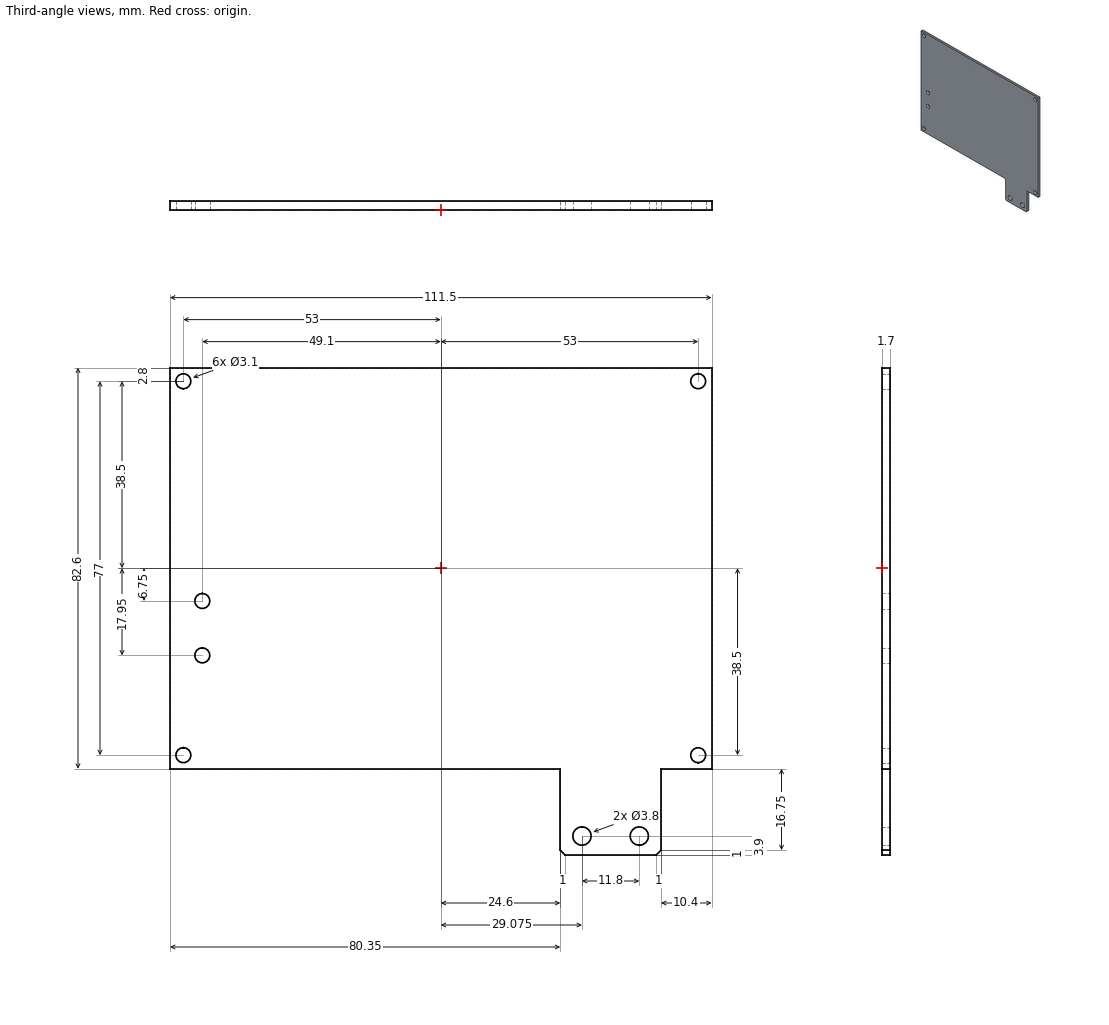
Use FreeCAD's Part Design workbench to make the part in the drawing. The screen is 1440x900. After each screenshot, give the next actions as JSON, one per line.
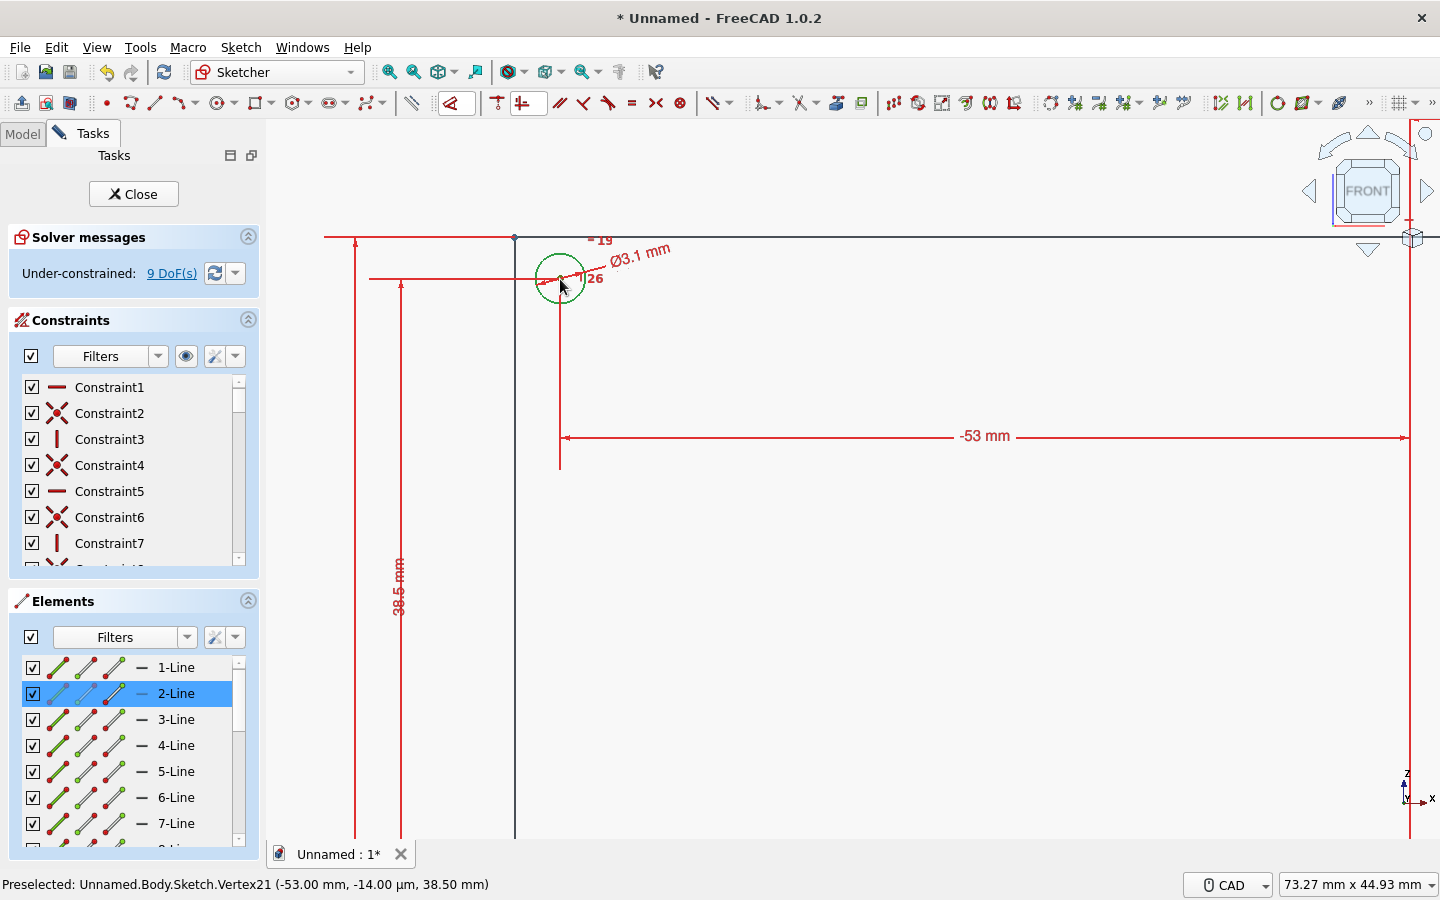
{"action": "key", "text": "i"}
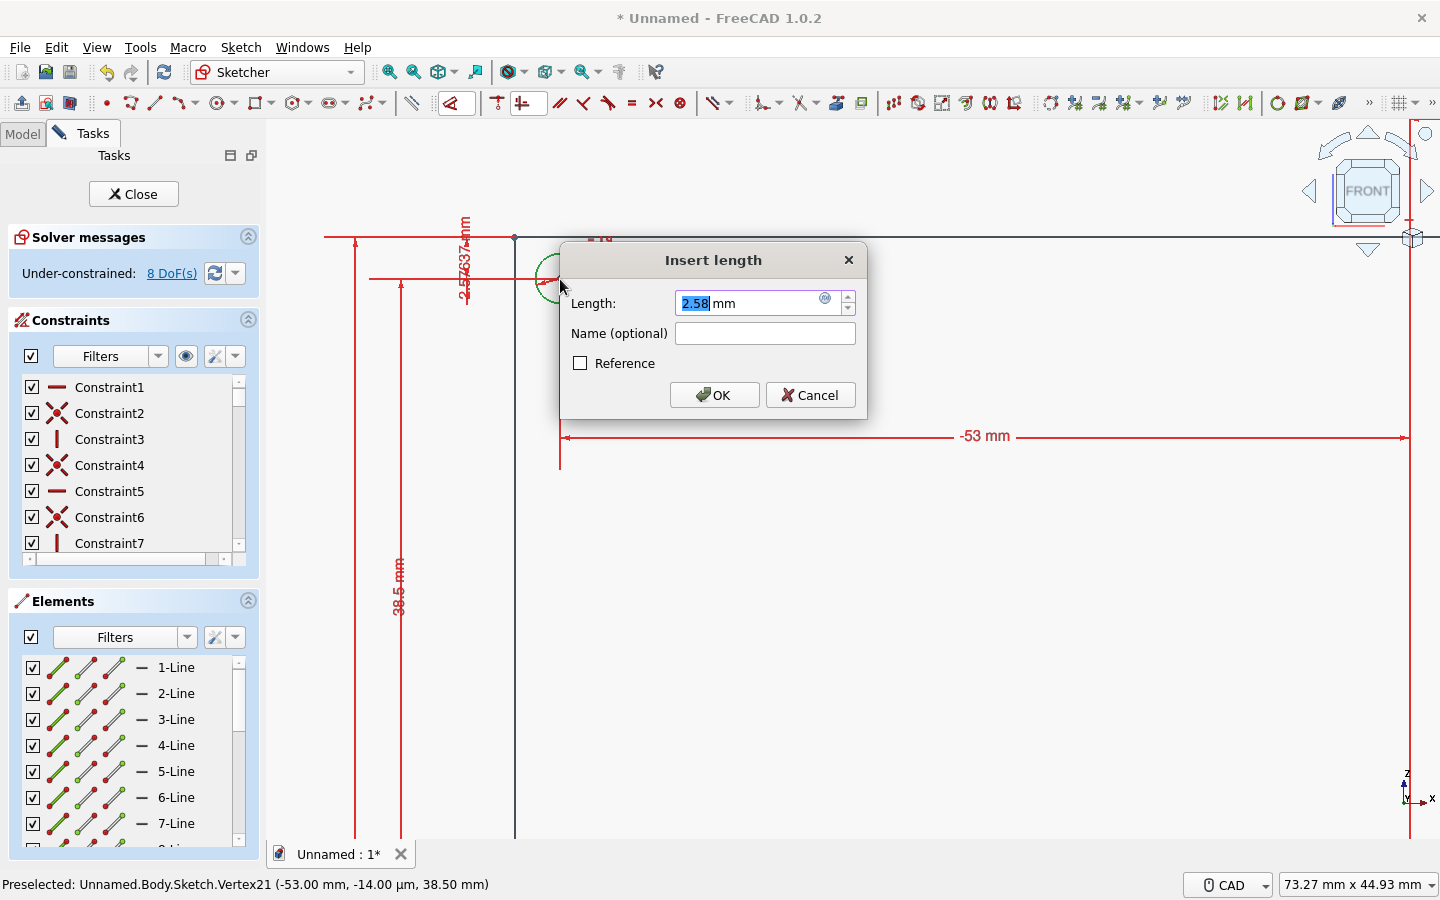
{"action": "type", "text": "2.8"}
{"action": "key", "text": "Return"}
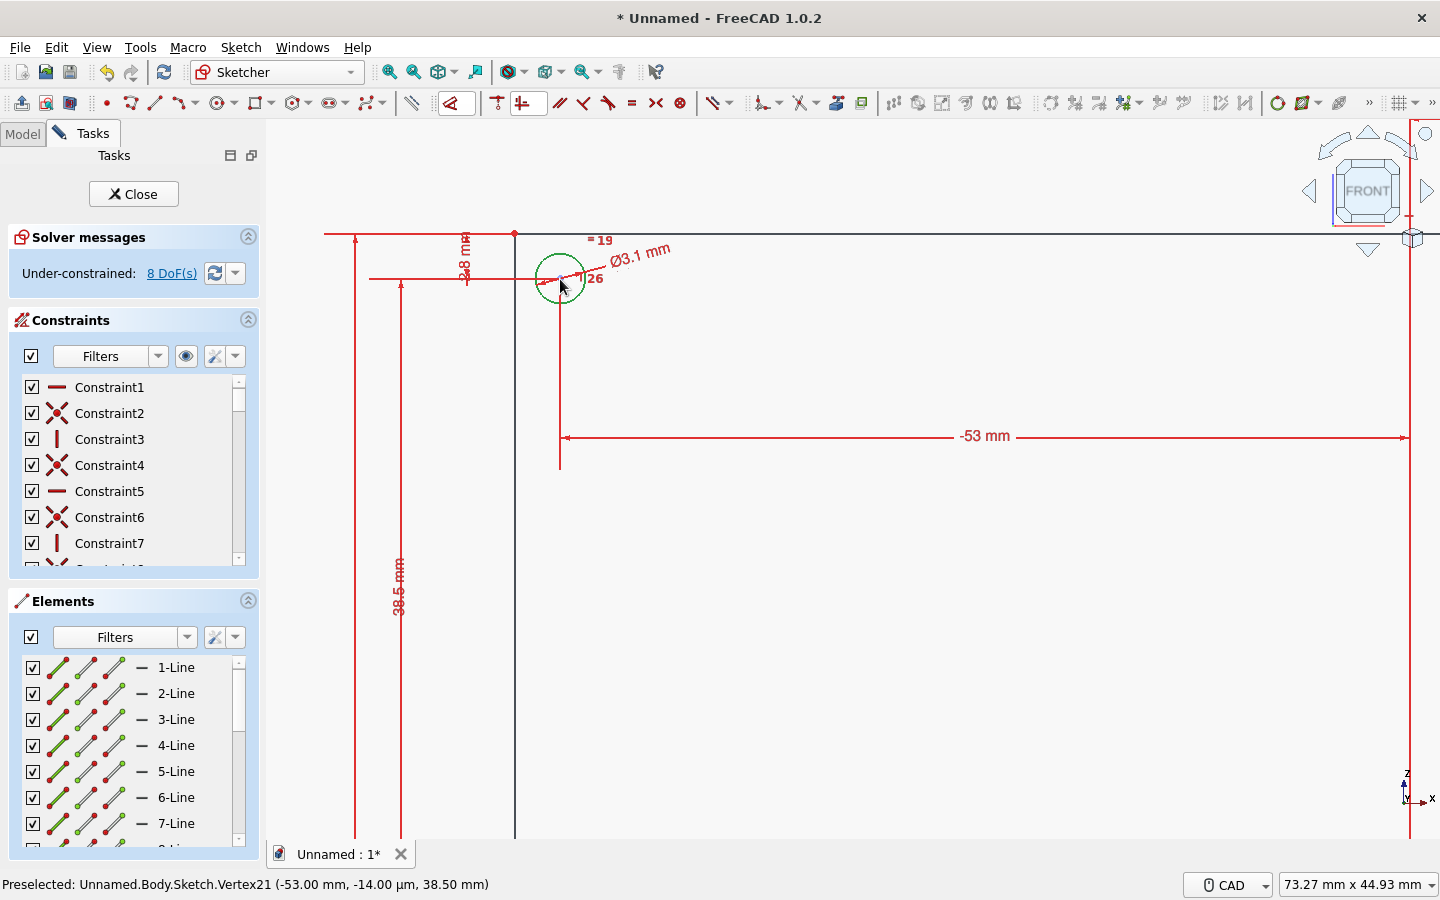
{"action": "scroll", "coordinate": [515, 238], "scroll_direction": "down", "scroll_amount": 6}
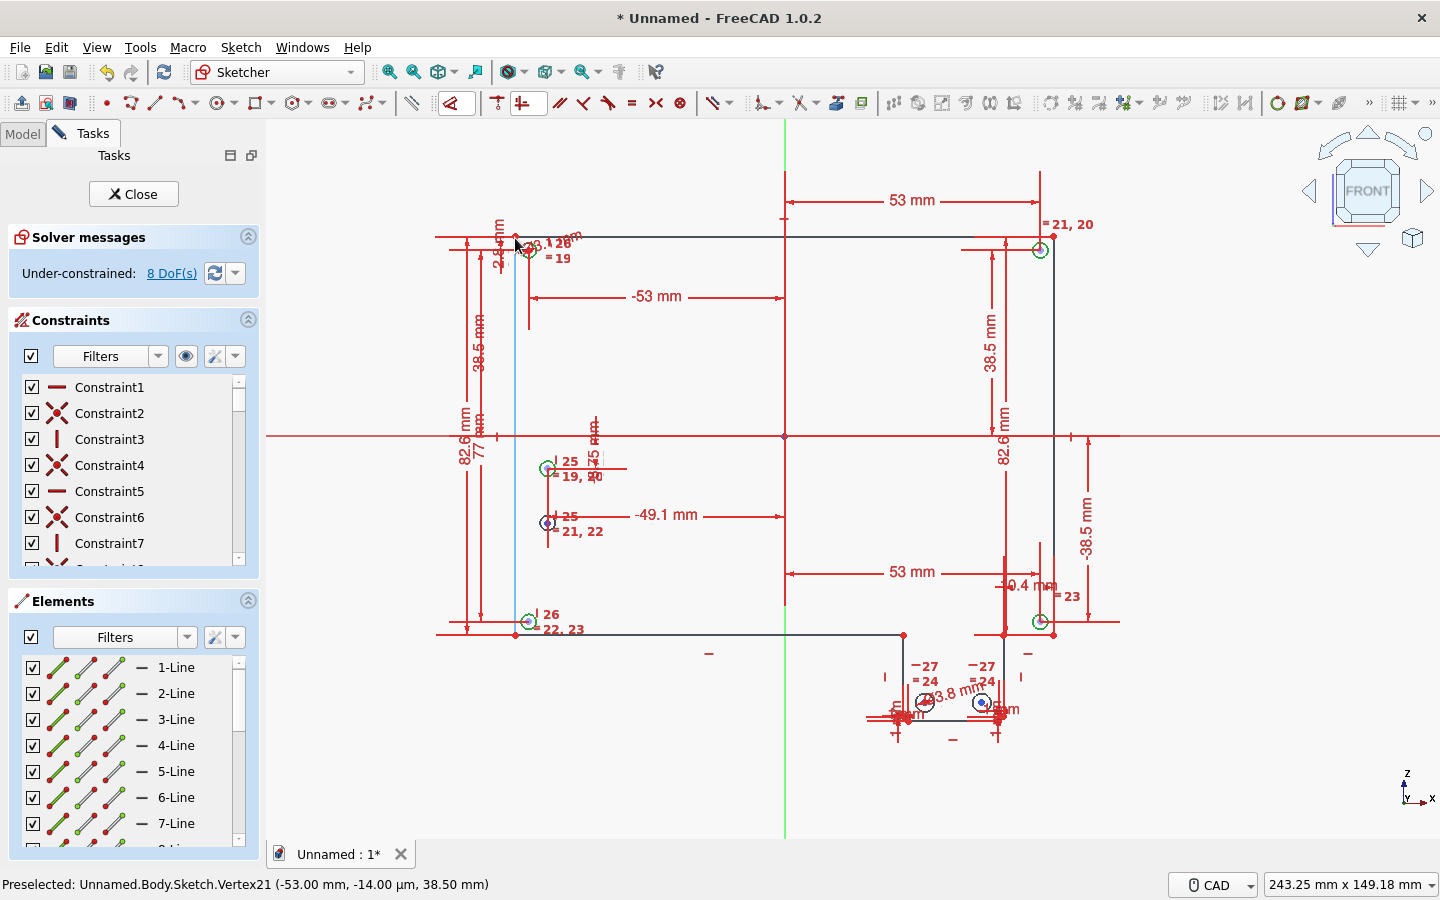
{"action": "scroll", "coordinate": [908, 721], "scroll_direction": "up", "scroll_amount": 4}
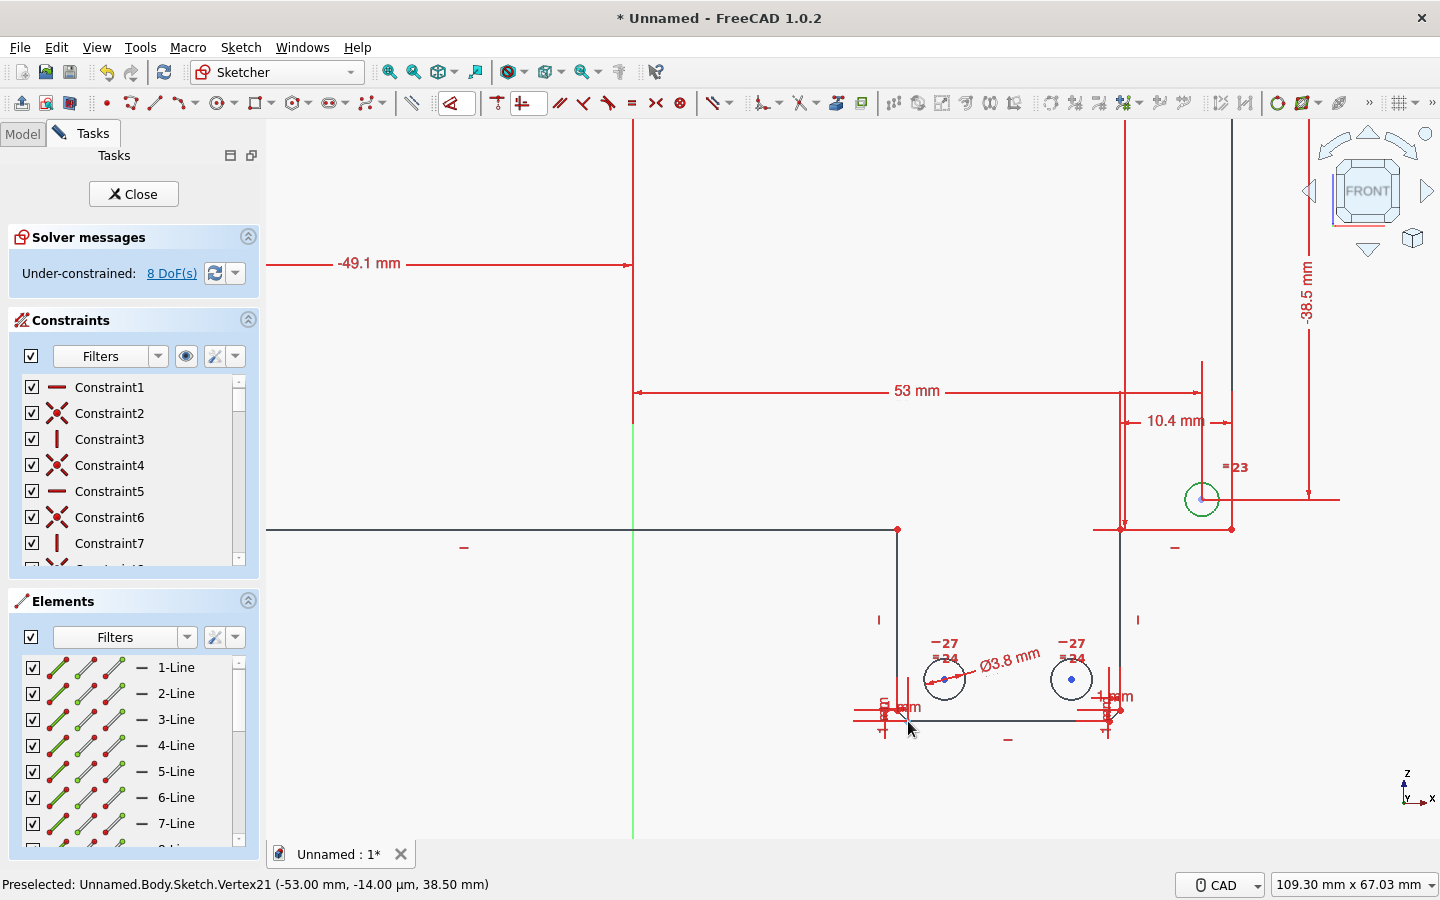
{"action": "left_click", "coordinate": [908, 721]}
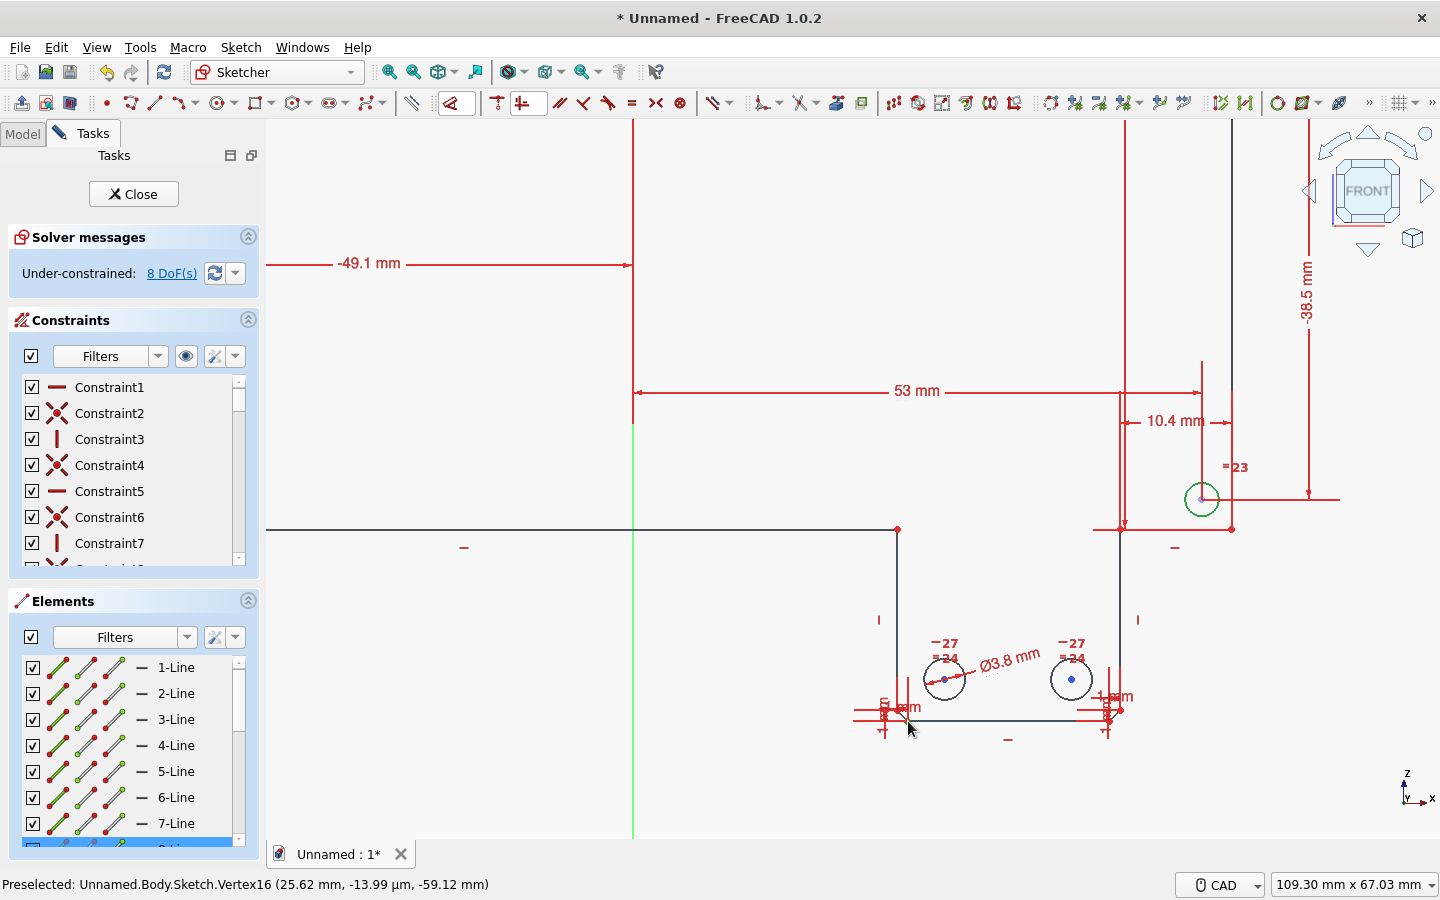
{"action": "left_click", "coordinate": [945, 679]}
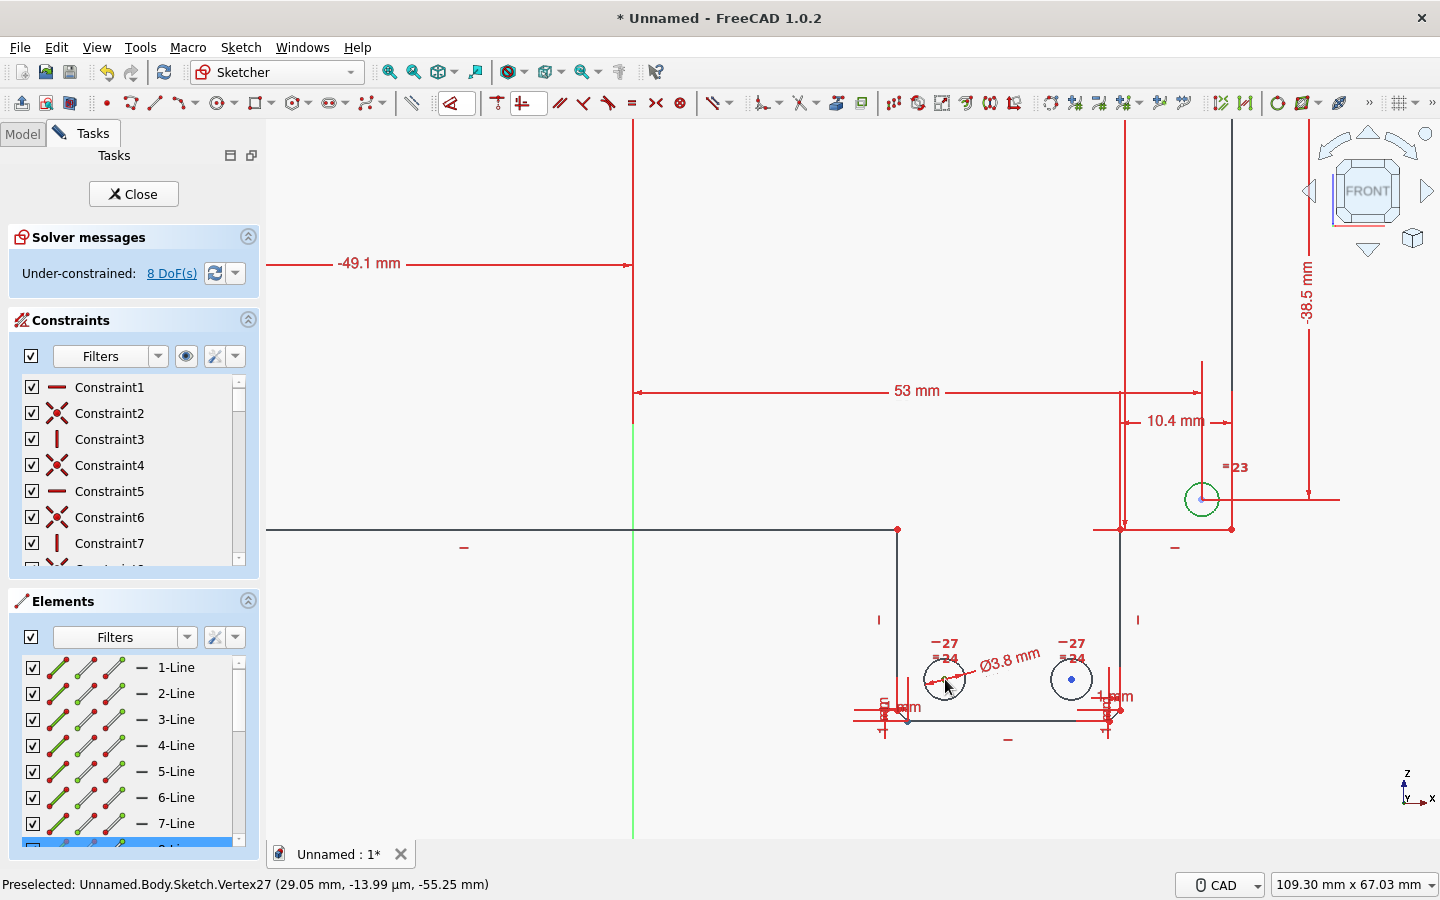
{"action": "key", "text": "i"}